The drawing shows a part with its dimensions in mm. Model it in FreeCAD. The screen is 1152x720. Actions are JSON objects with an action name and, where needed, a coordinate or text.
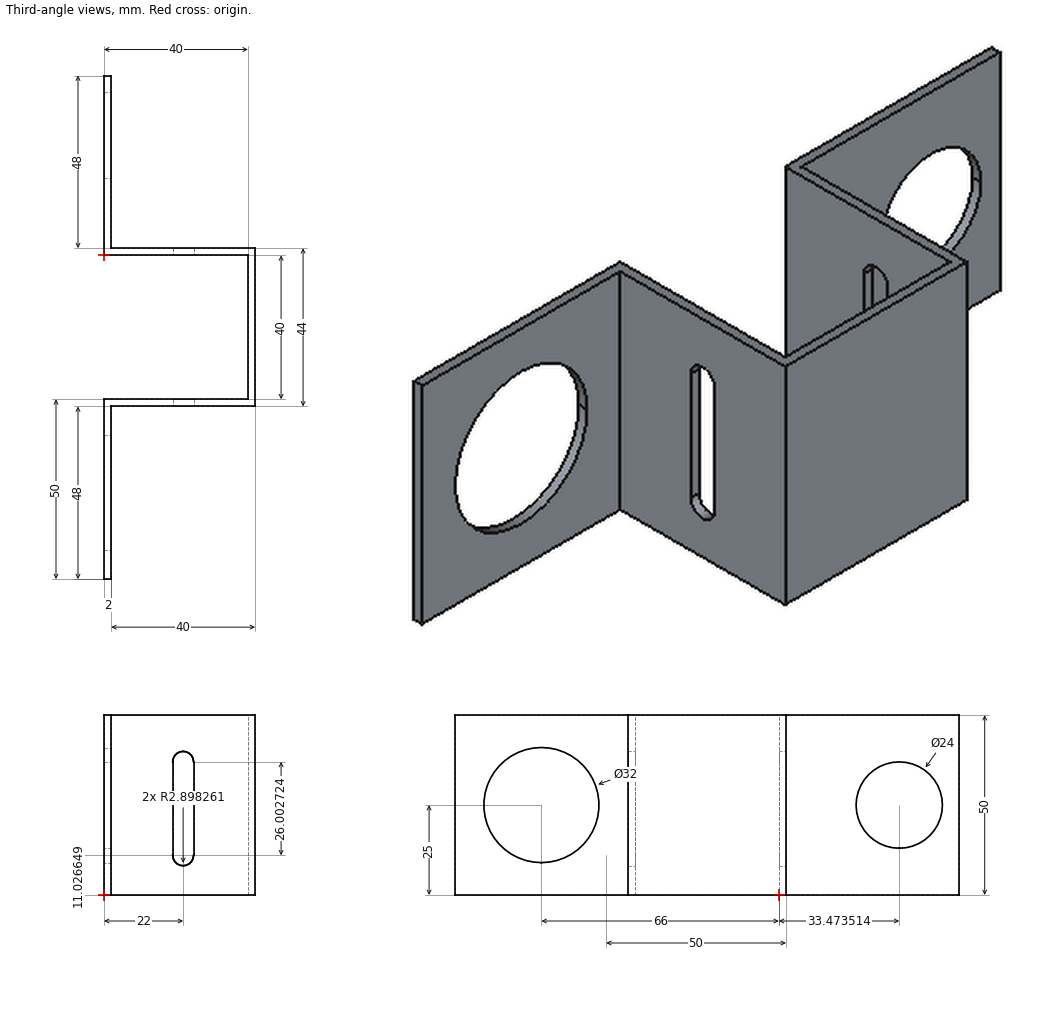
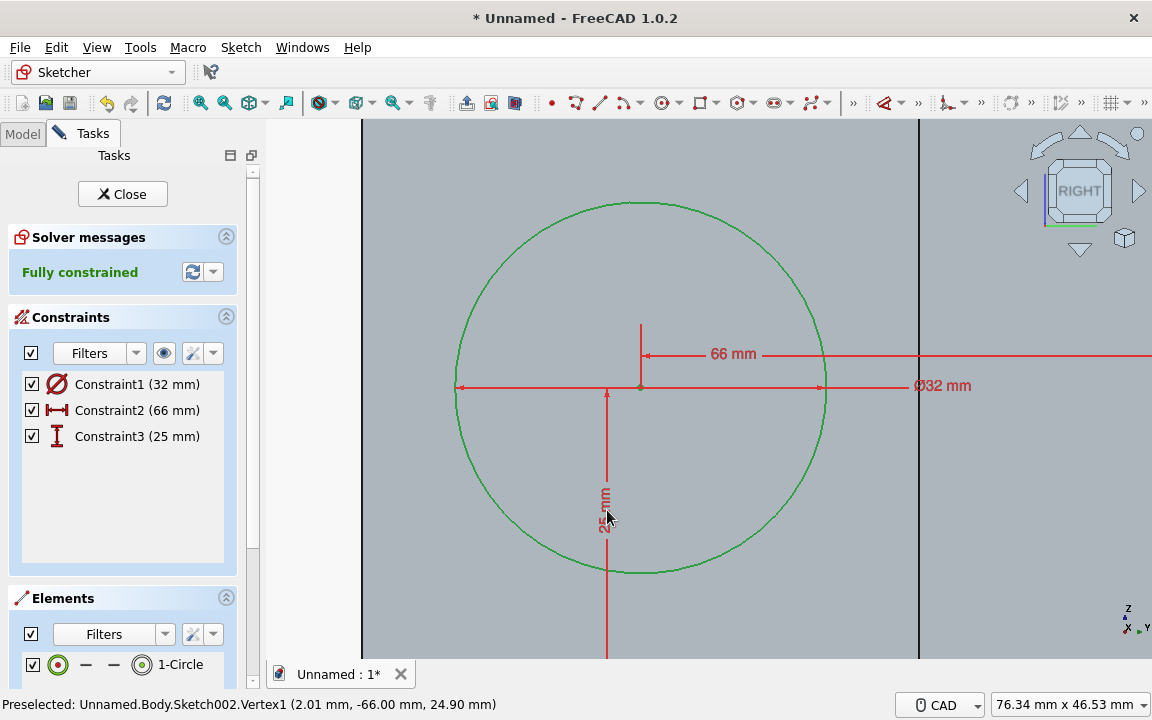
{"action": "left_click", "coordinate": [123, 194]}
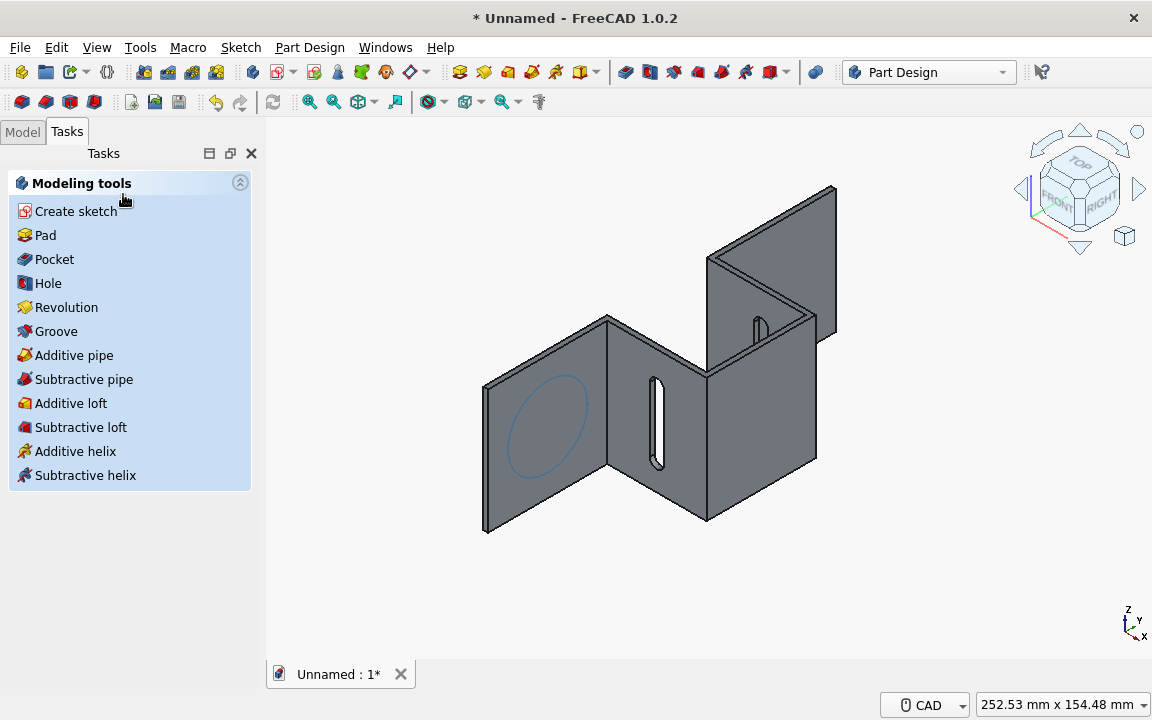
{"action": "left_click", "coordinate": [626, 72]}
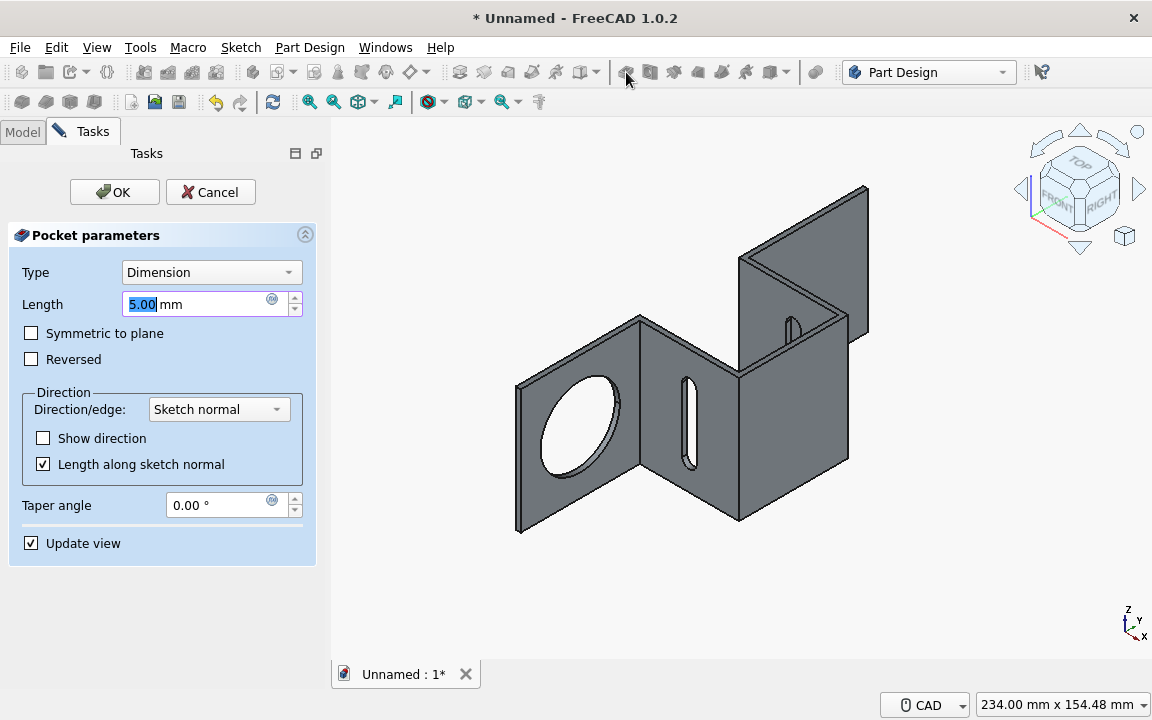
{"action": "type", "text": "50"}
{"action": "key", "text": "Tab"}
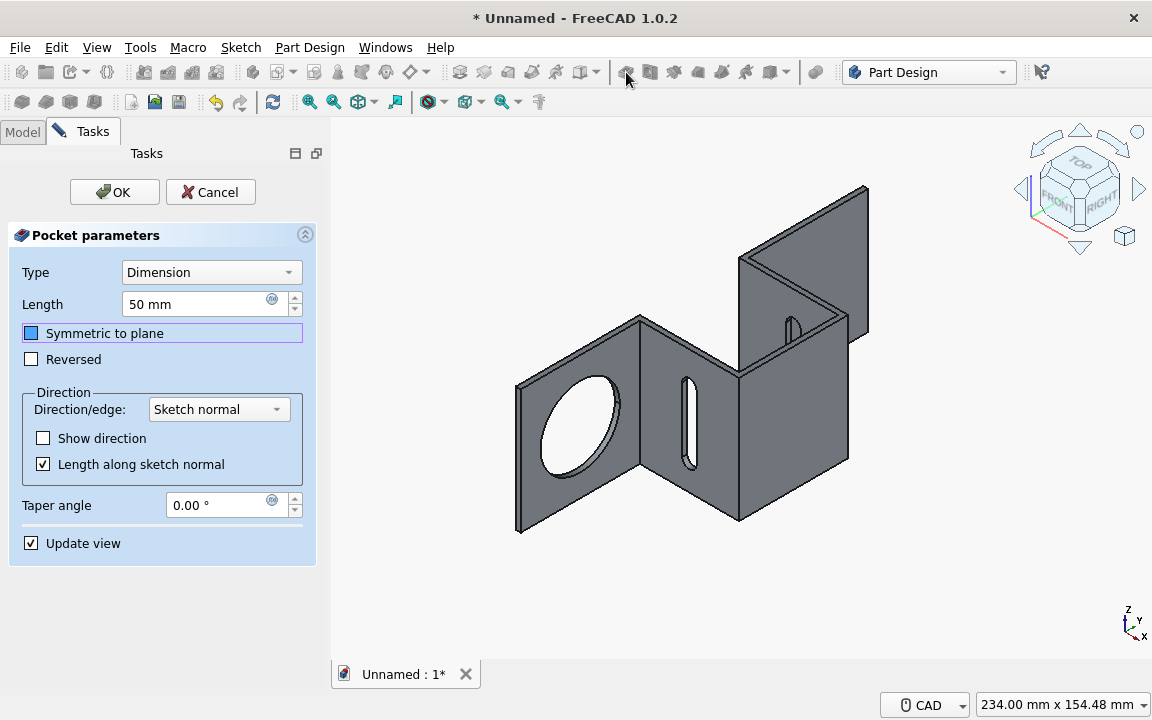
{"action": "left_click", "coordinate": [115, 192]}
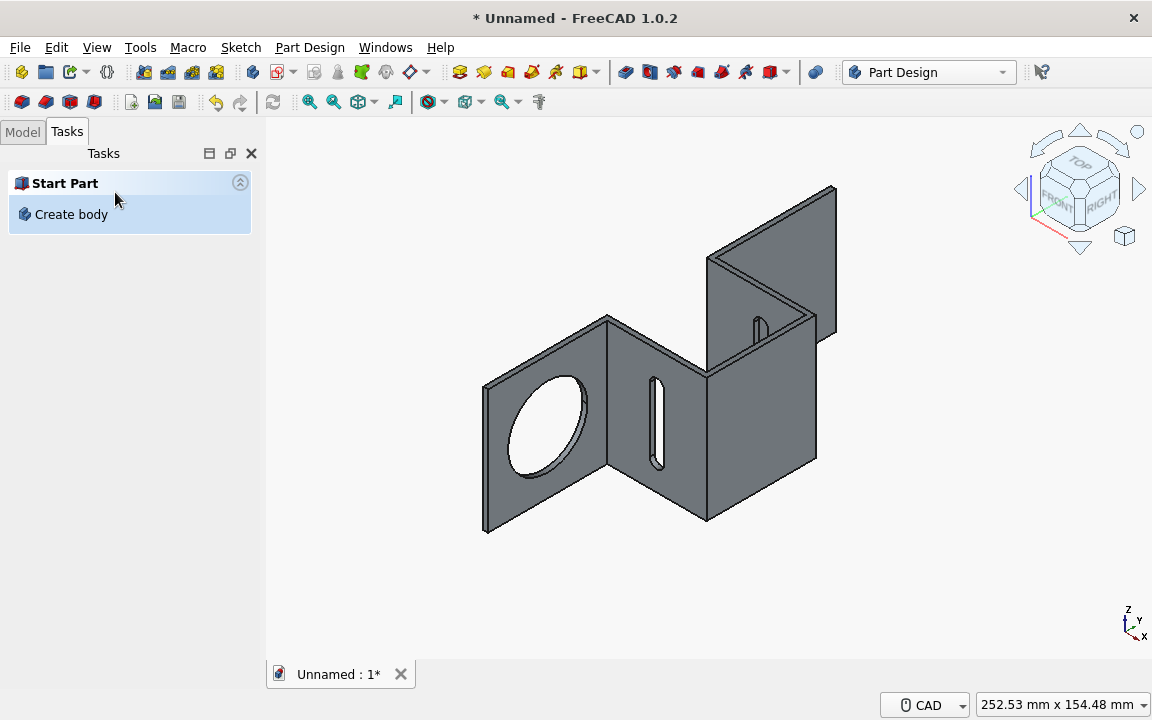
{"action": "left_click", "coordinate": [776, 273]}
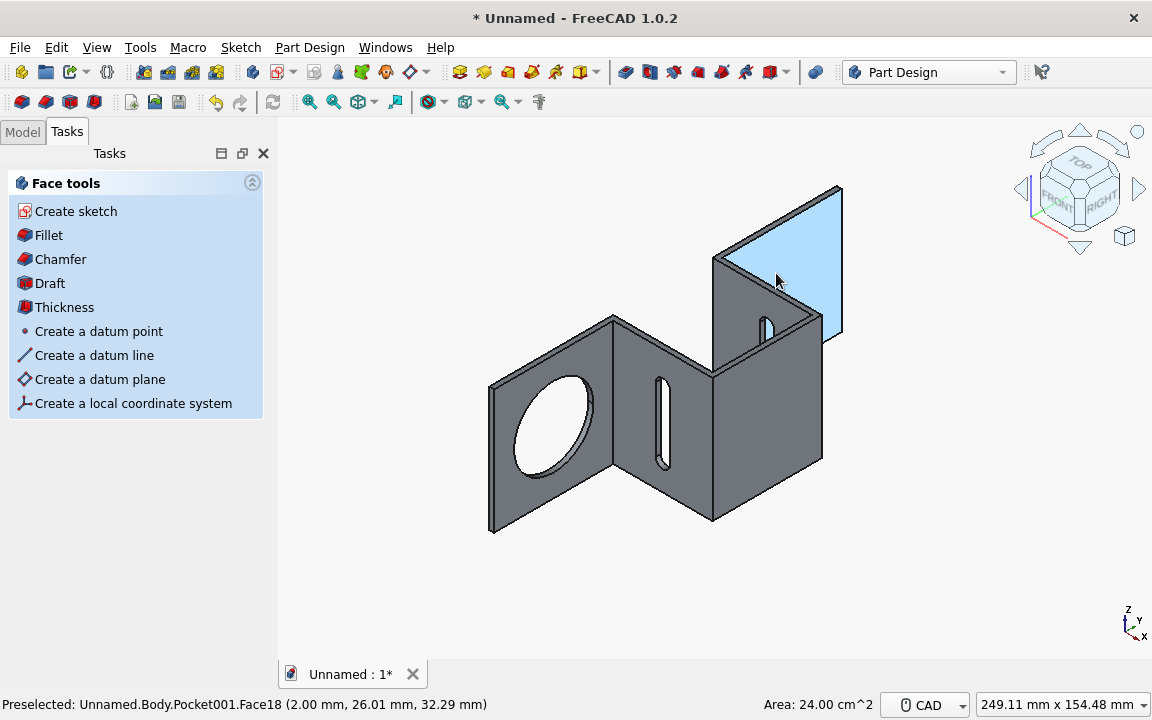
{"action": "left_click", "coordinate": [278, 72]}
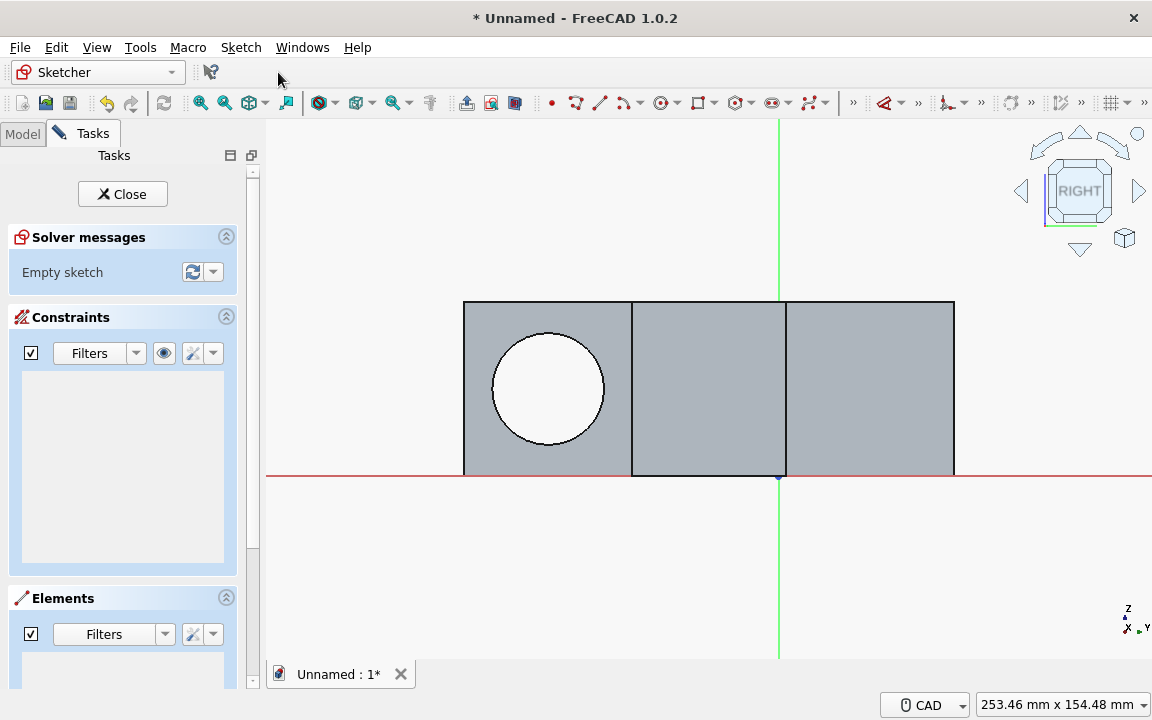
{"action": "scroll", "coordinate": [985, 425], "scroll_direction": "up", "scroll_amount": 5}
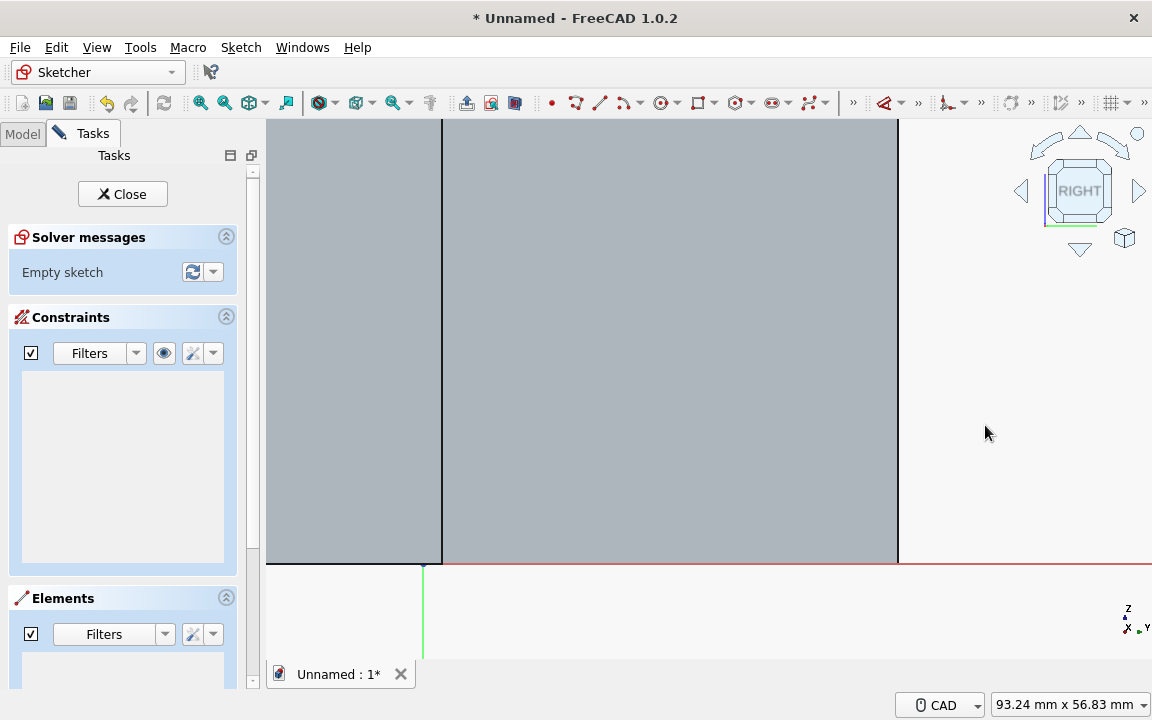
{"action": "left_click", "coordinate": [662, 104]}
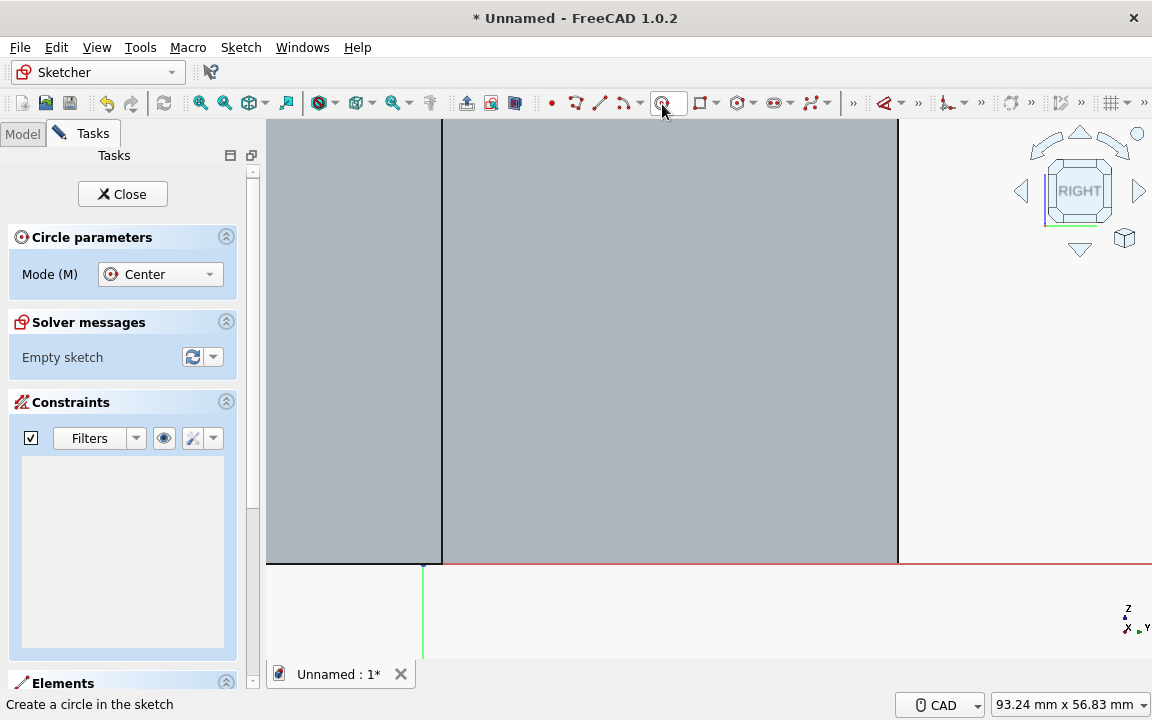
{"action": "left_click", "coordinate": [741, 326]}
{"action": "mouse_move", "coordinate": [822, 246]}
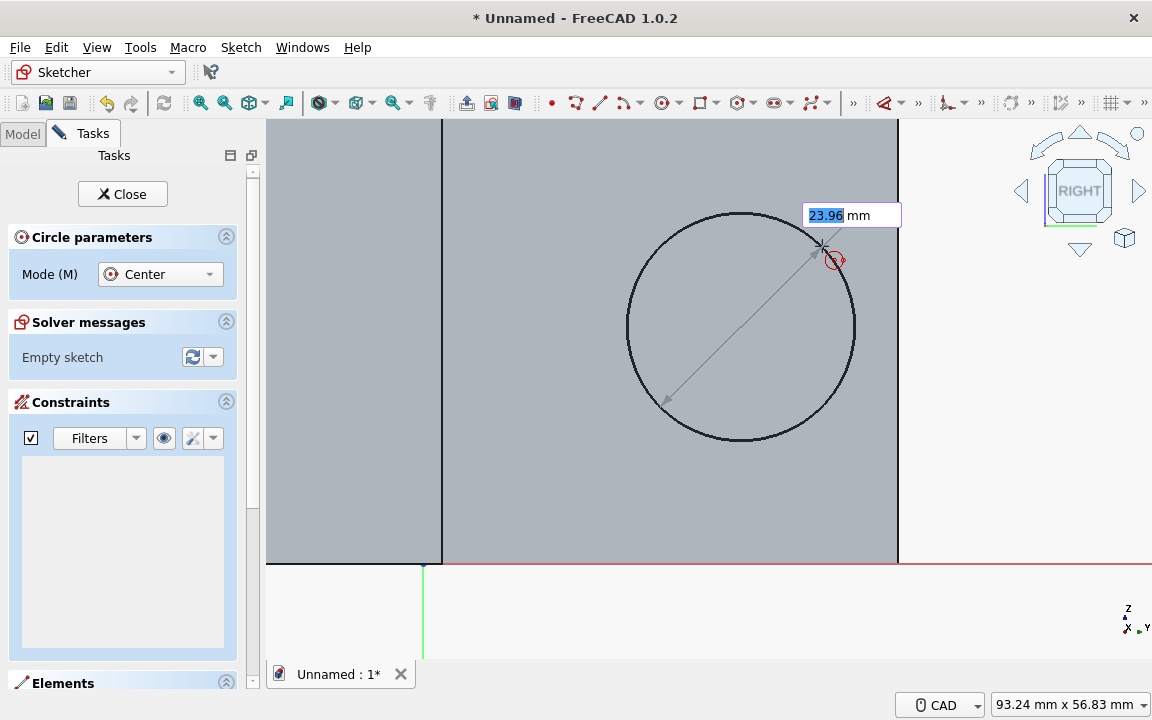
{"action": "type", "text": "24"}
{"action": "key", "text": "Return"}
{"action": "key", "text": "Escape"}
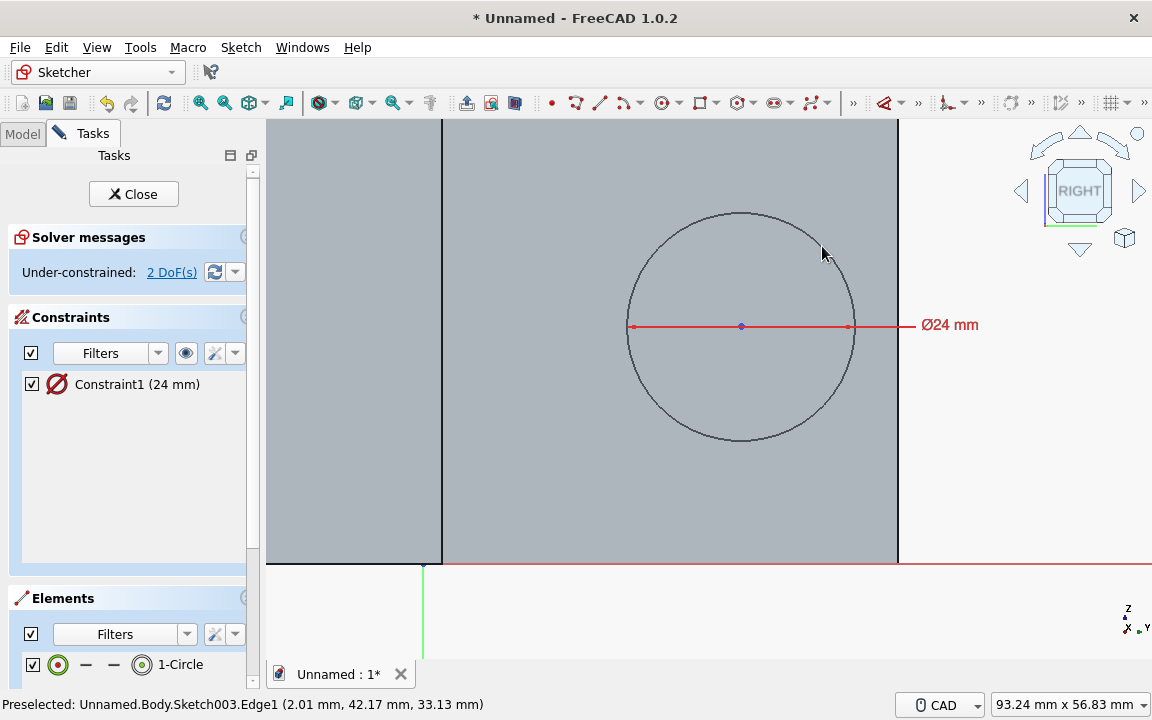
{"action": "left_click", "coordinate": [884, 104]}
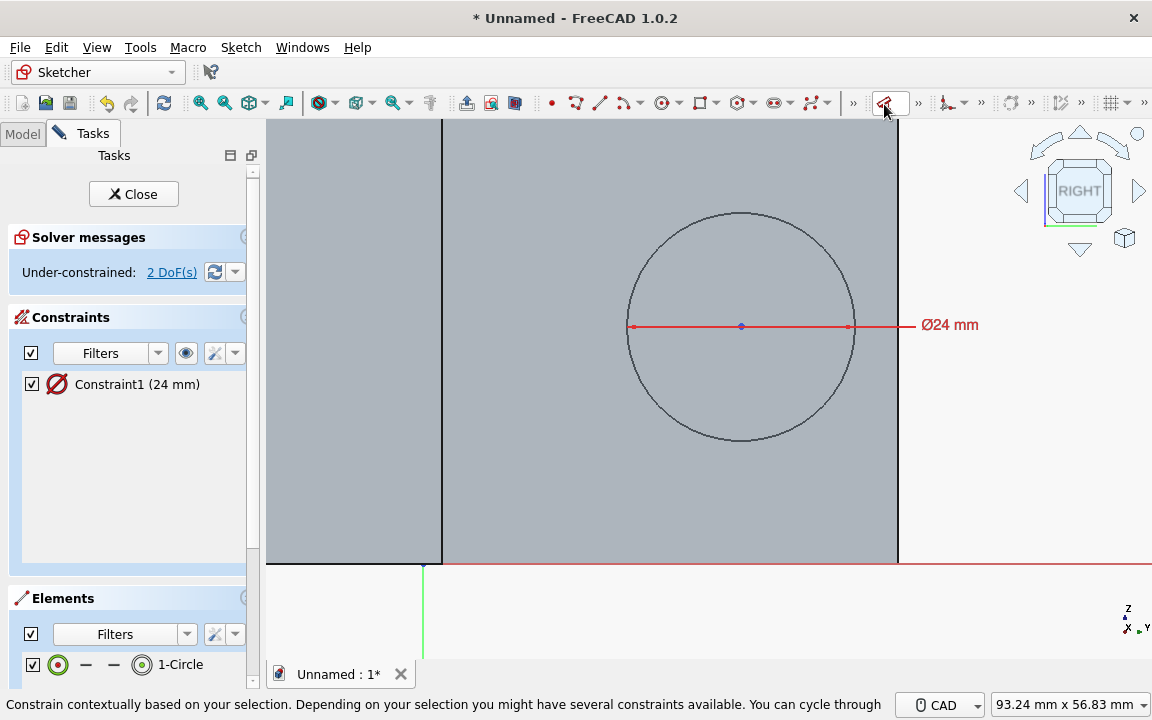
{"action": "left_click", "coordinate": [741, 327]}
{"action": "left_click", "coordinate": [389, 445]}